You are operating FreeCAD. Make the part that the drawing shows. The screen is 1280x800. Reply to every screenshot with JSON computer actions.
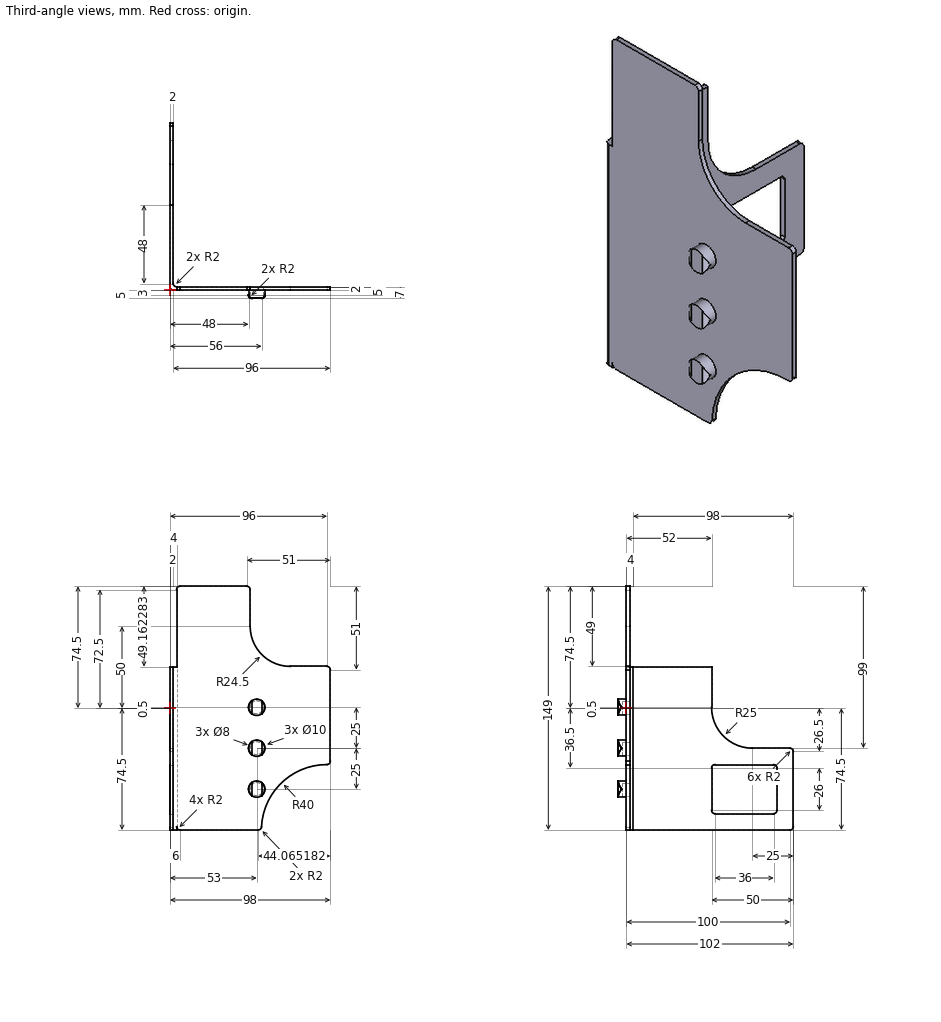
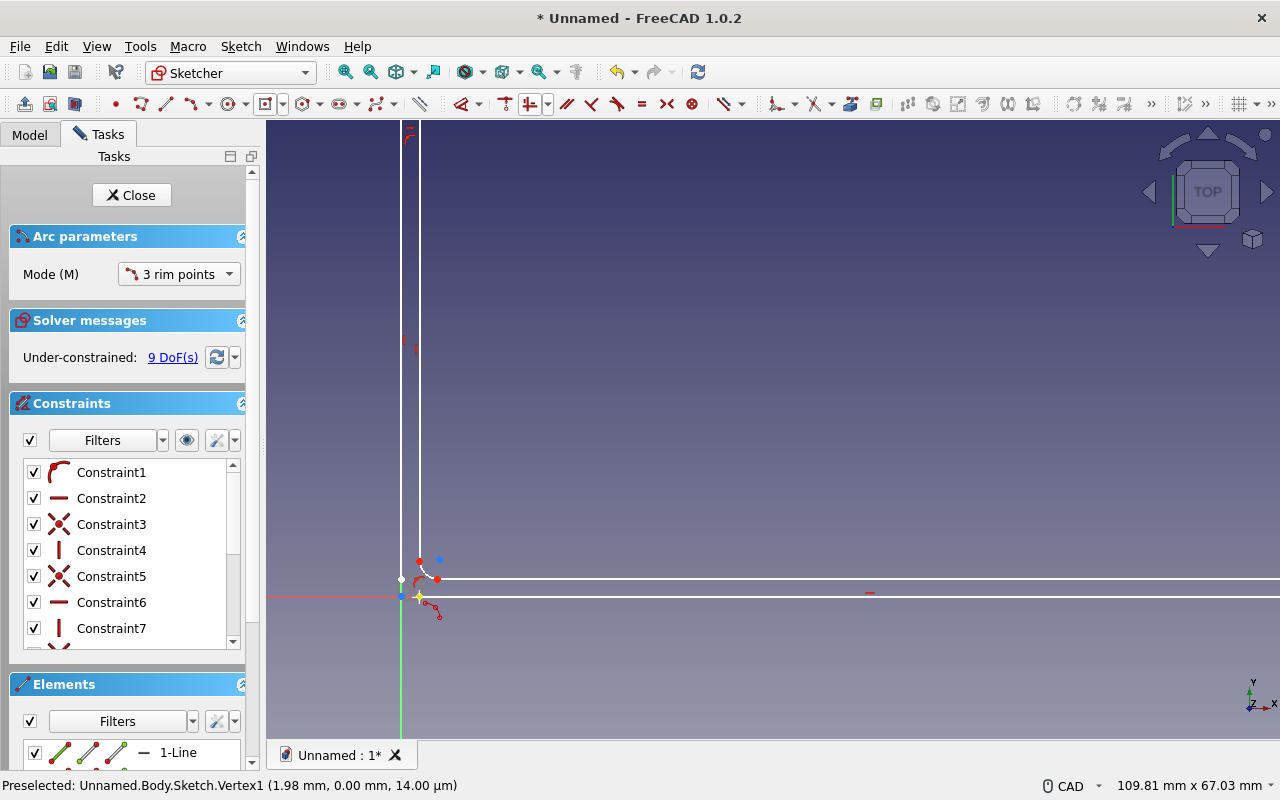
{"action": "scroll", "coordinate": [406, 591], "scroll_direction": "up", "scroll_amount": 6}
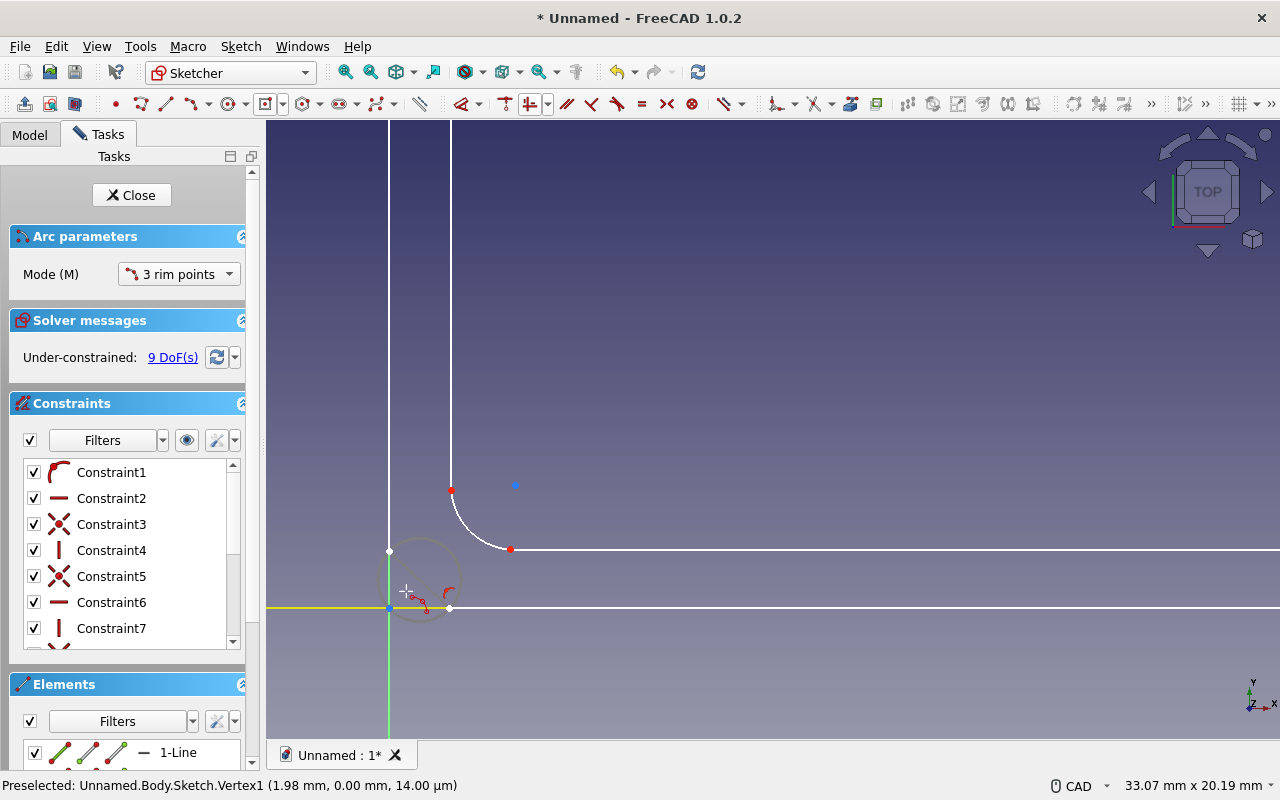
{"action": "left_click", "coordinate": [407, 591]}
{"action": "key", "text": "Escape"}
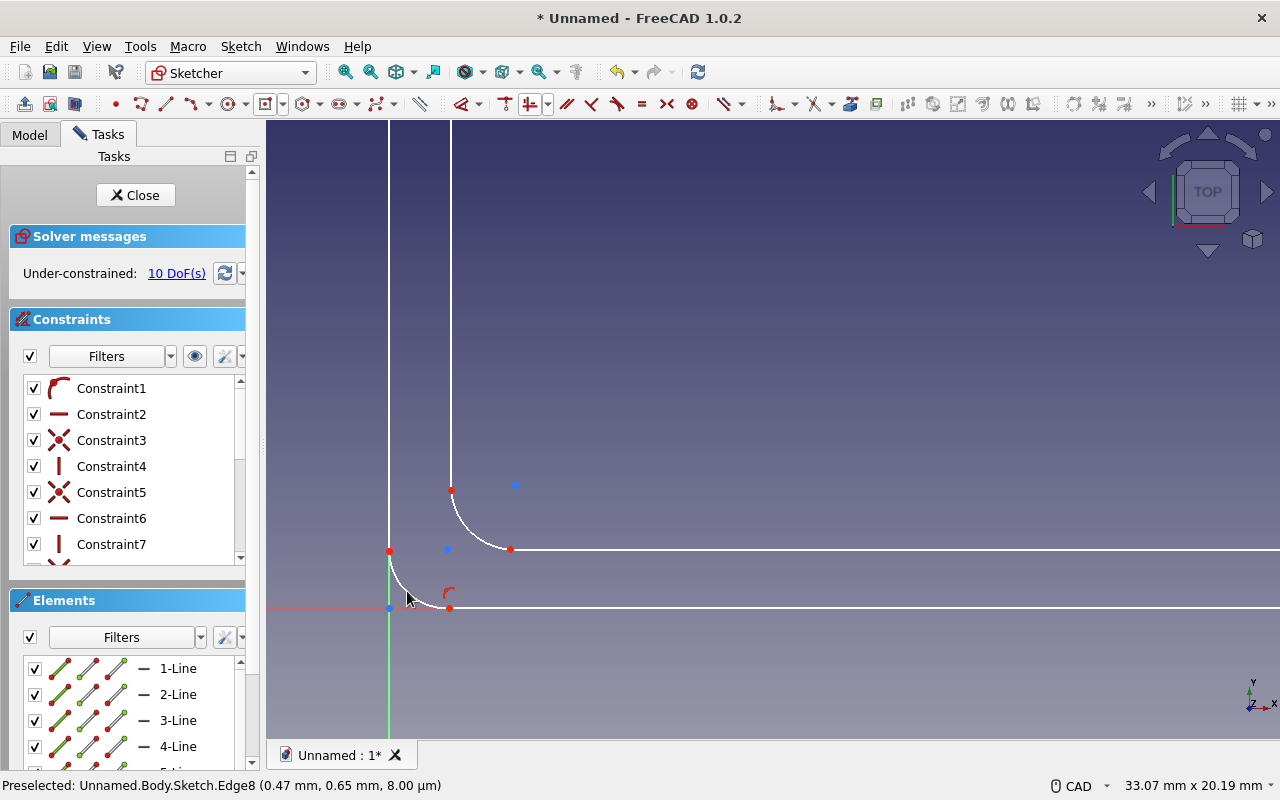
{"action": "scroll", "coordinate": [404, 586], "scroll_direction": "down", "scroll_amount": 8}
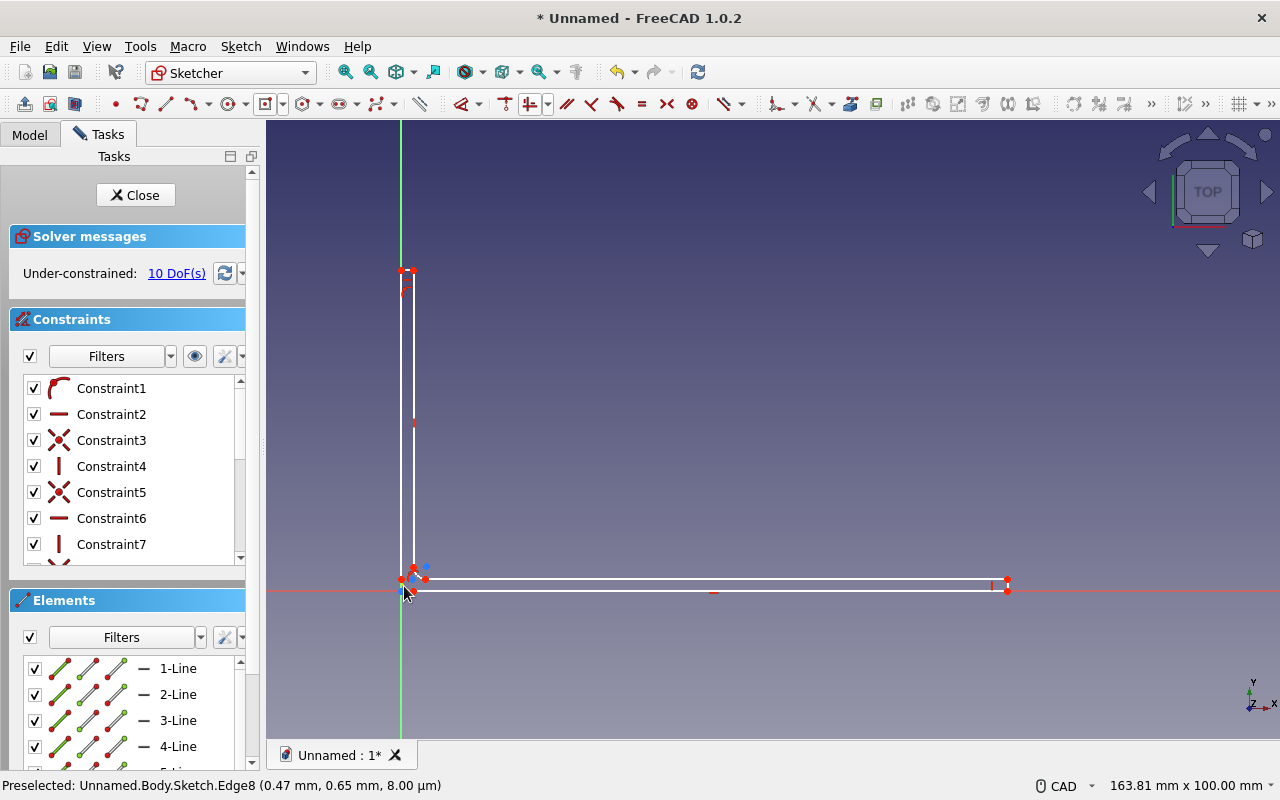
{"action": "left_click", "coordinate": [532, 591]}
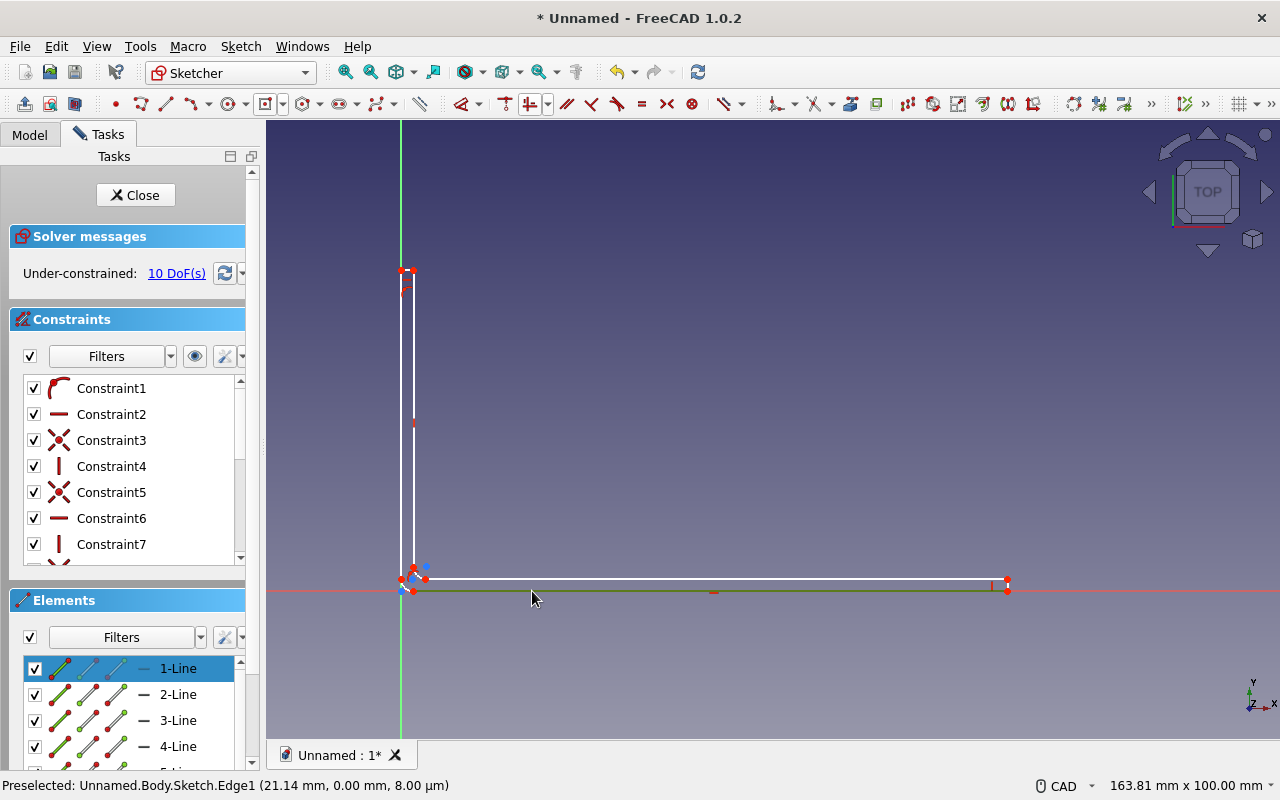
{"action": "scroll", "coordinate": [405, 588], "scroll_direction": "up", "scroll_amount": 3}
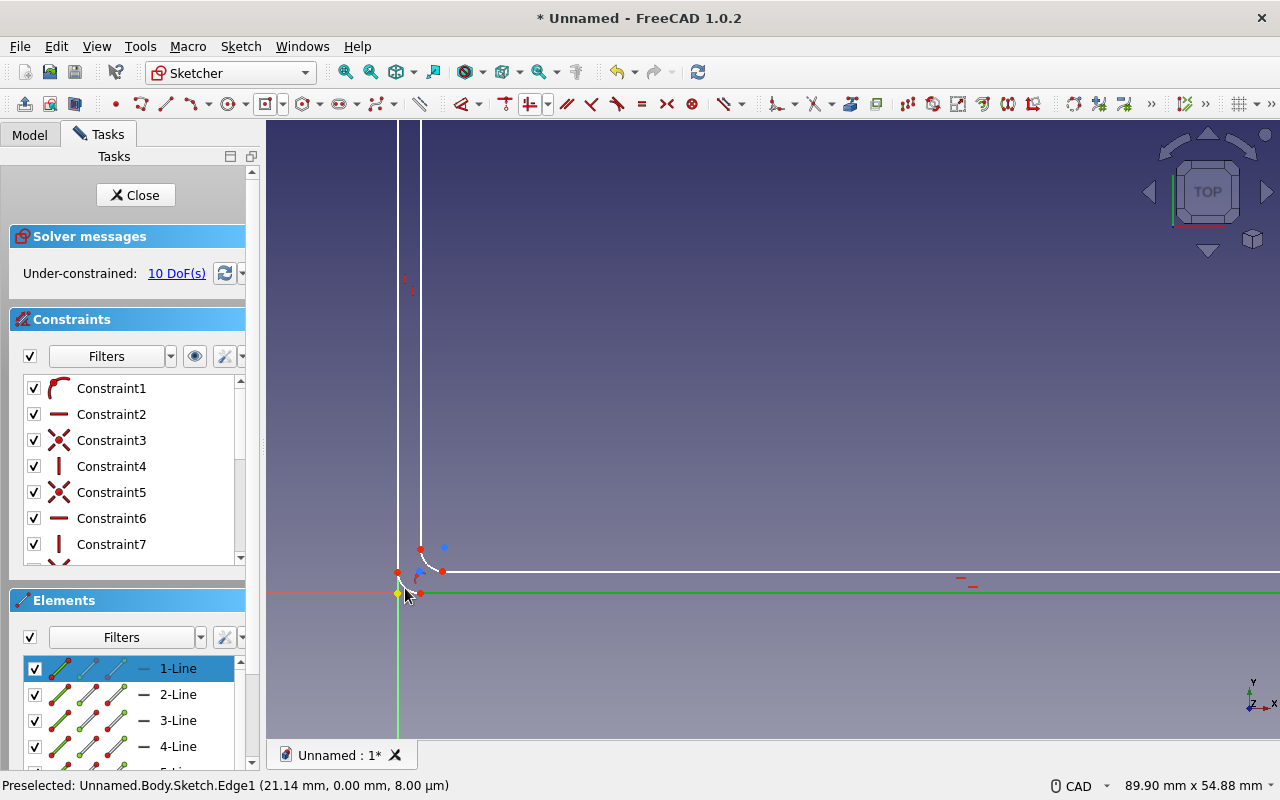
{"action": "left_click", "coordinate": [405, 587]}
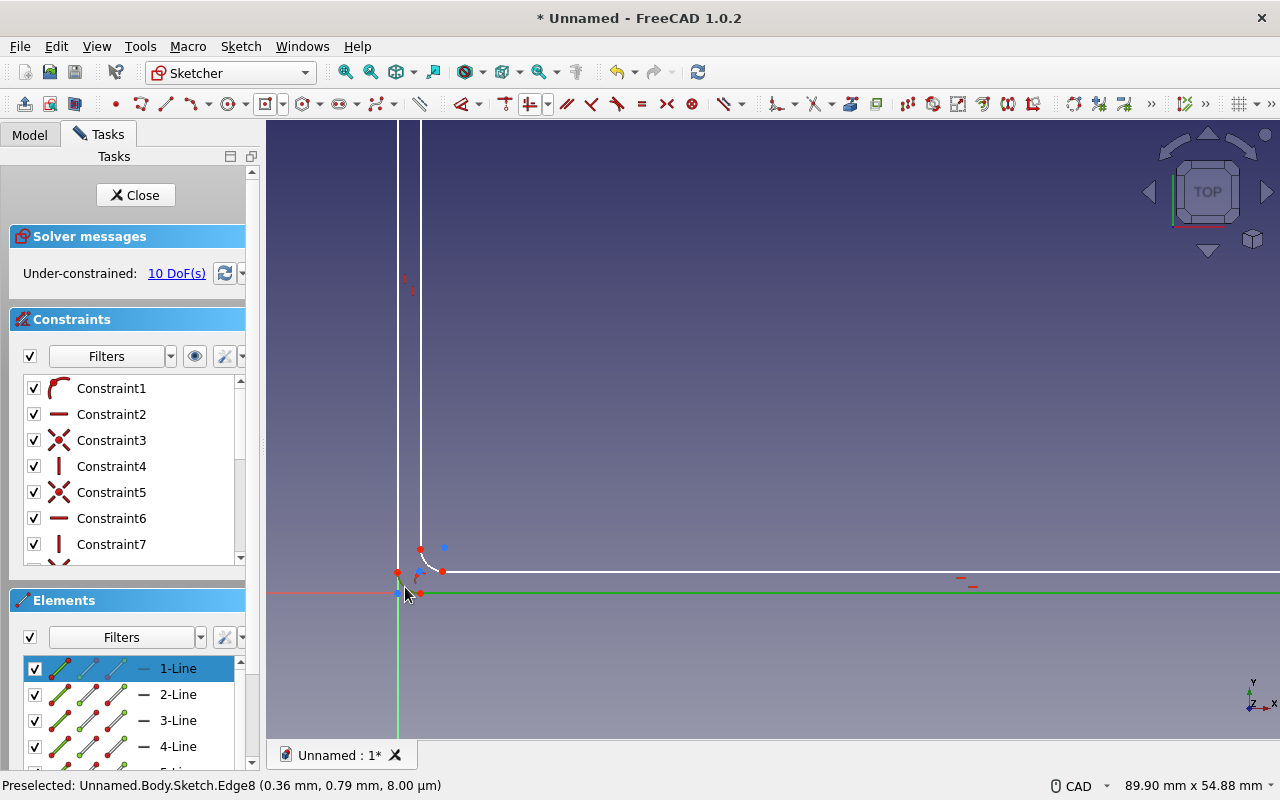
{"action": "key", "text": "t"}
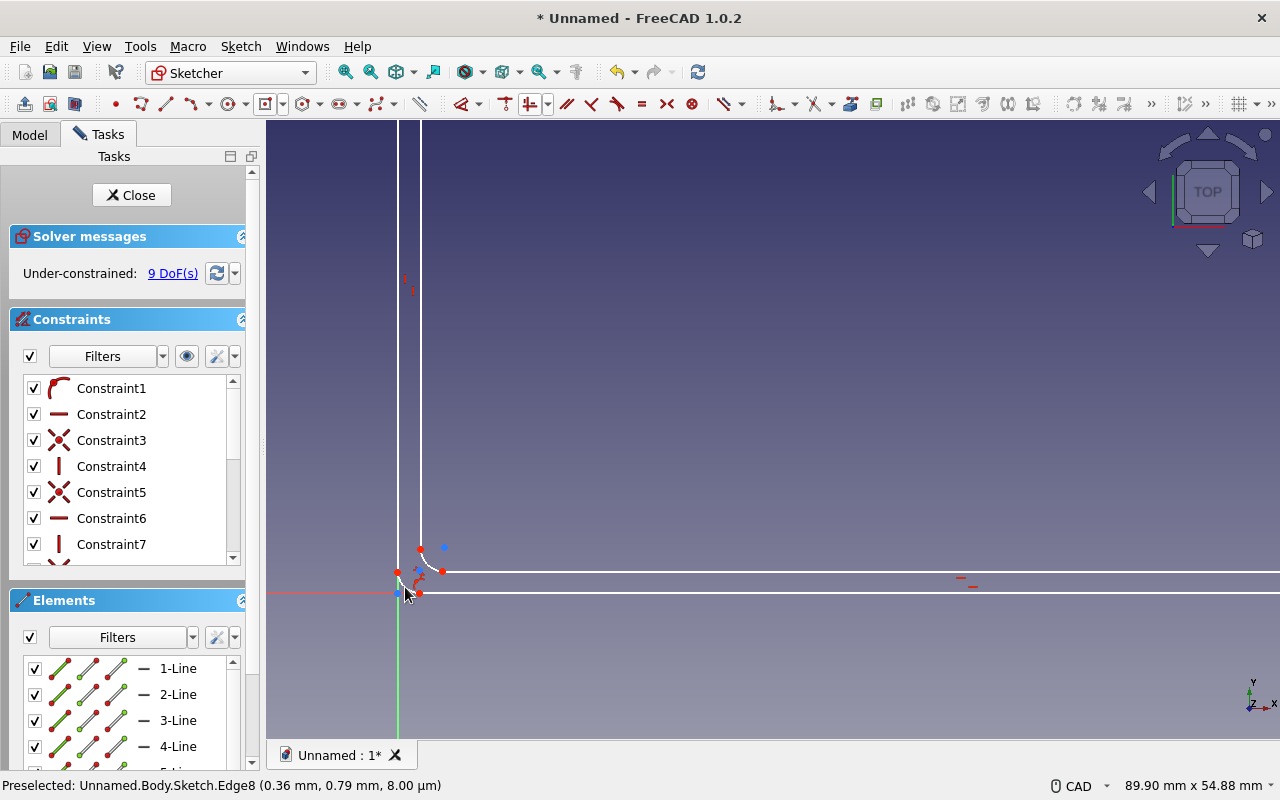
{"action": "left_click", "coordinate": [761, 572]}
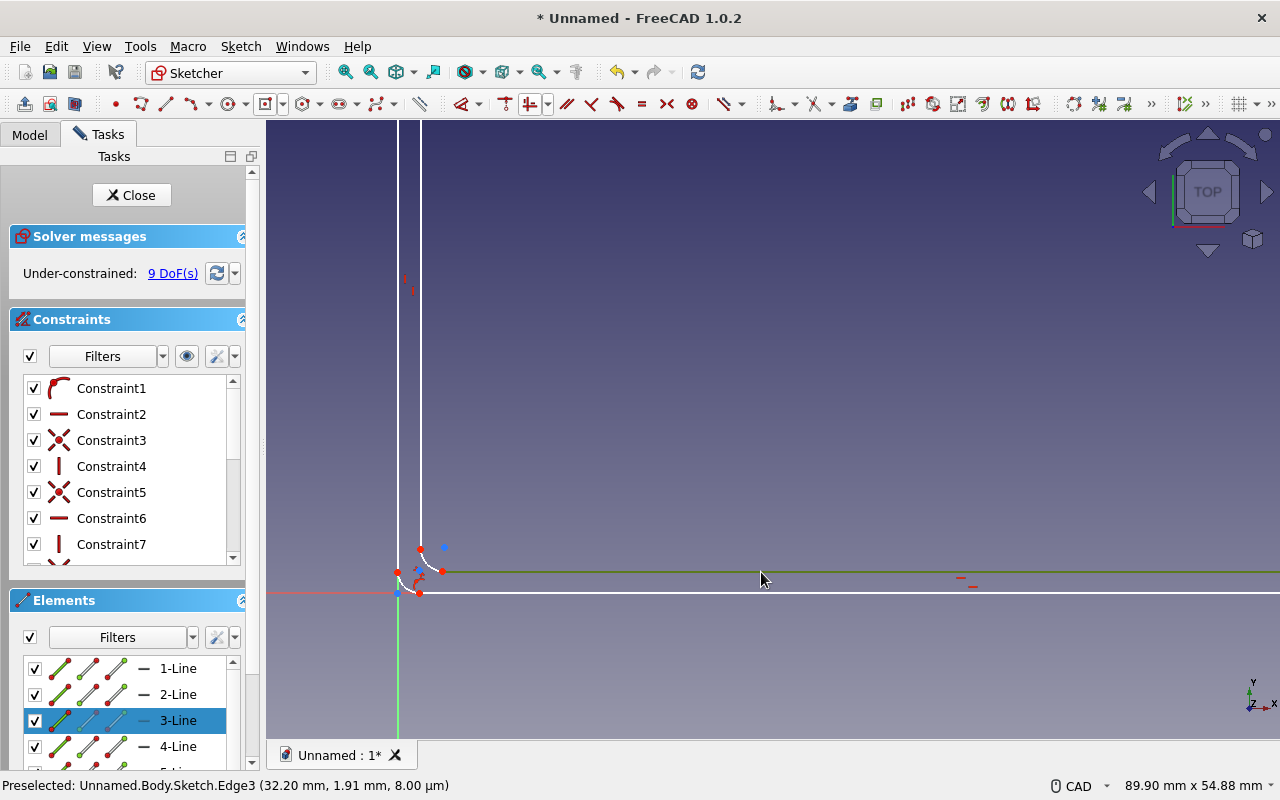
{"action": "scroll", "coordinate": [423, 559], "scroll_direction": "up", "scroll_amount": 2}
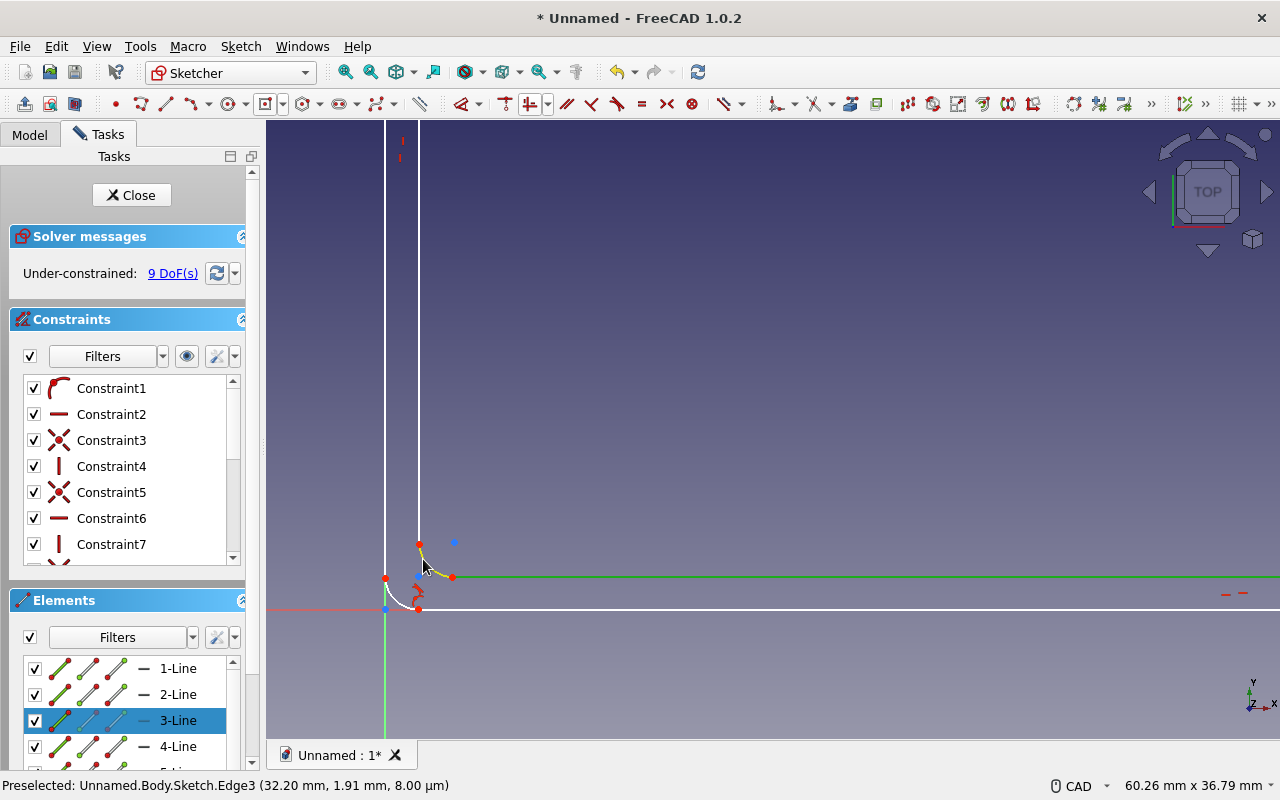
{"action": "left_click", "coordinate": [424, 559]}